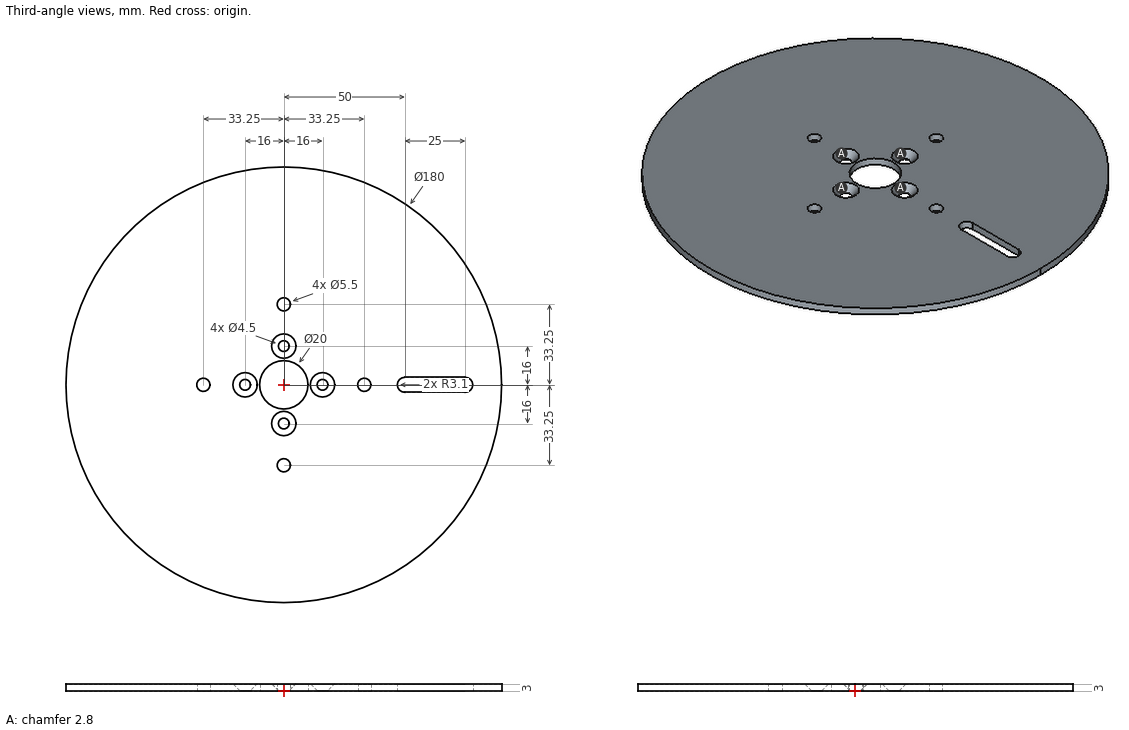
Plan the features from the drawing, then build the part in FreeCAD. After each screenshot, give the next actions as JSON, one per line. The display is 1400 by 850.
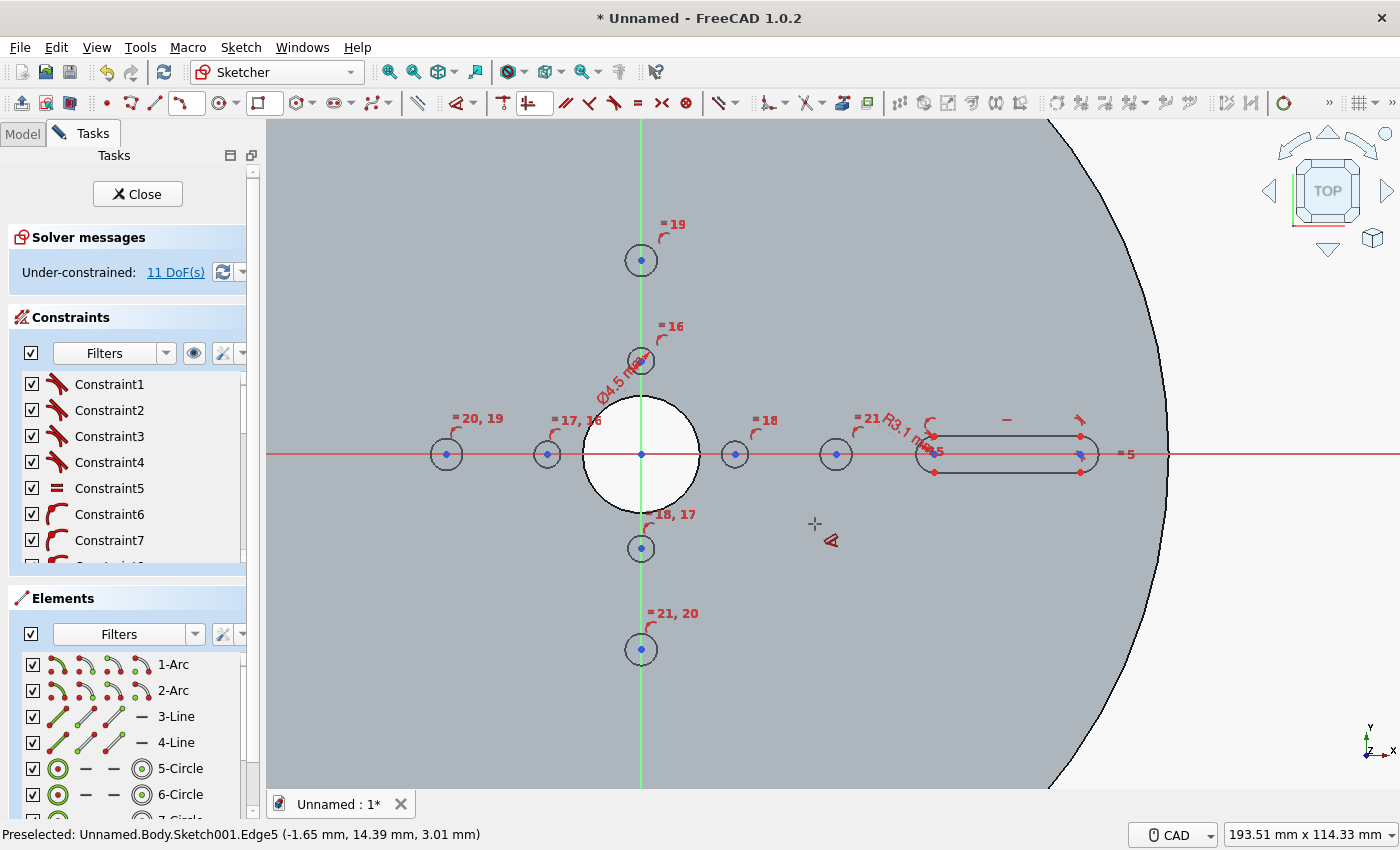
{"action": "scroll", "coordinate": [652, 249], "scroll_direction": "up", "scroll_amount": 2}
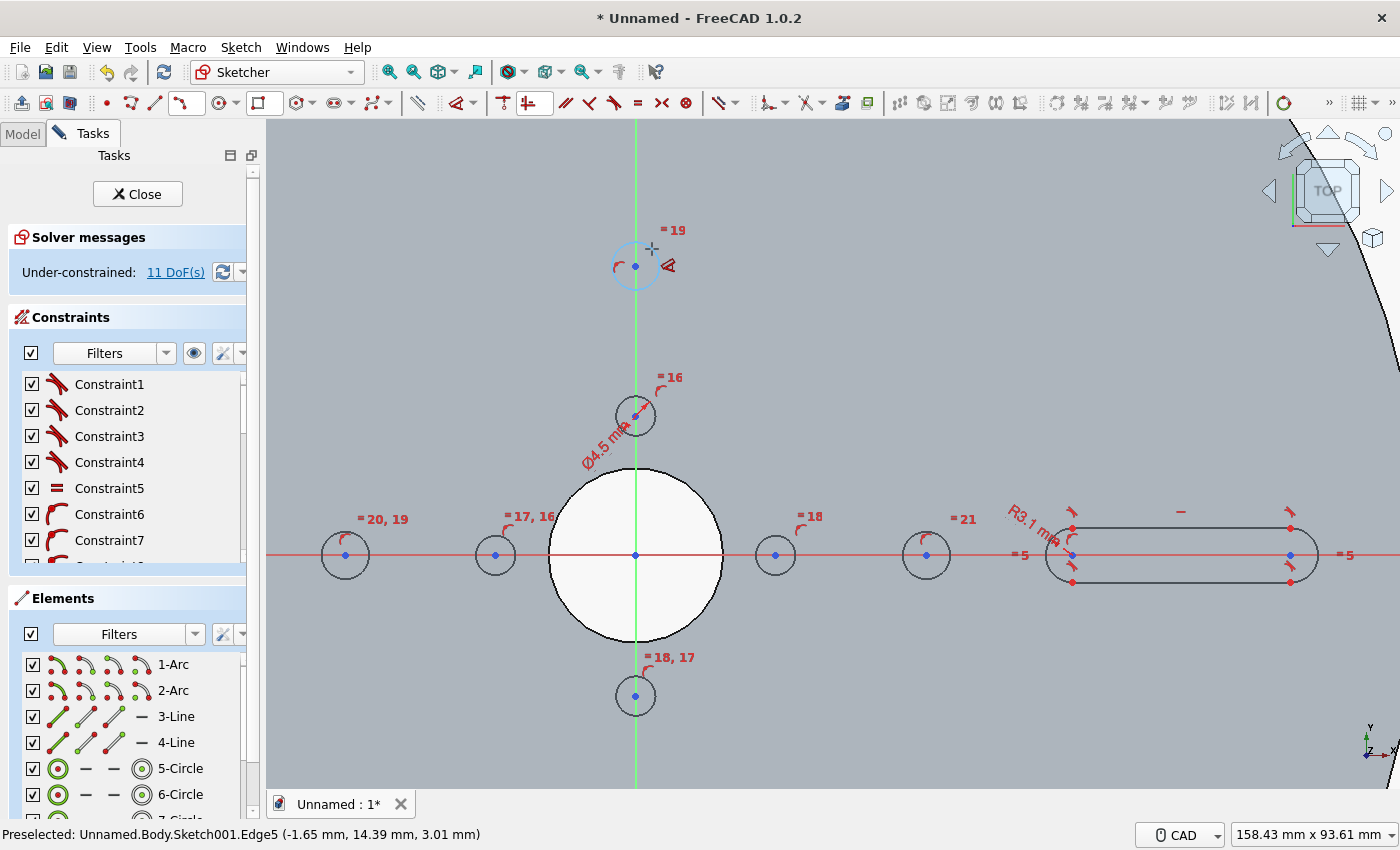
{"action": "left_click", "coordinate": [653, 249]}
{"action": "left_click", "coordinate": [676, 226]}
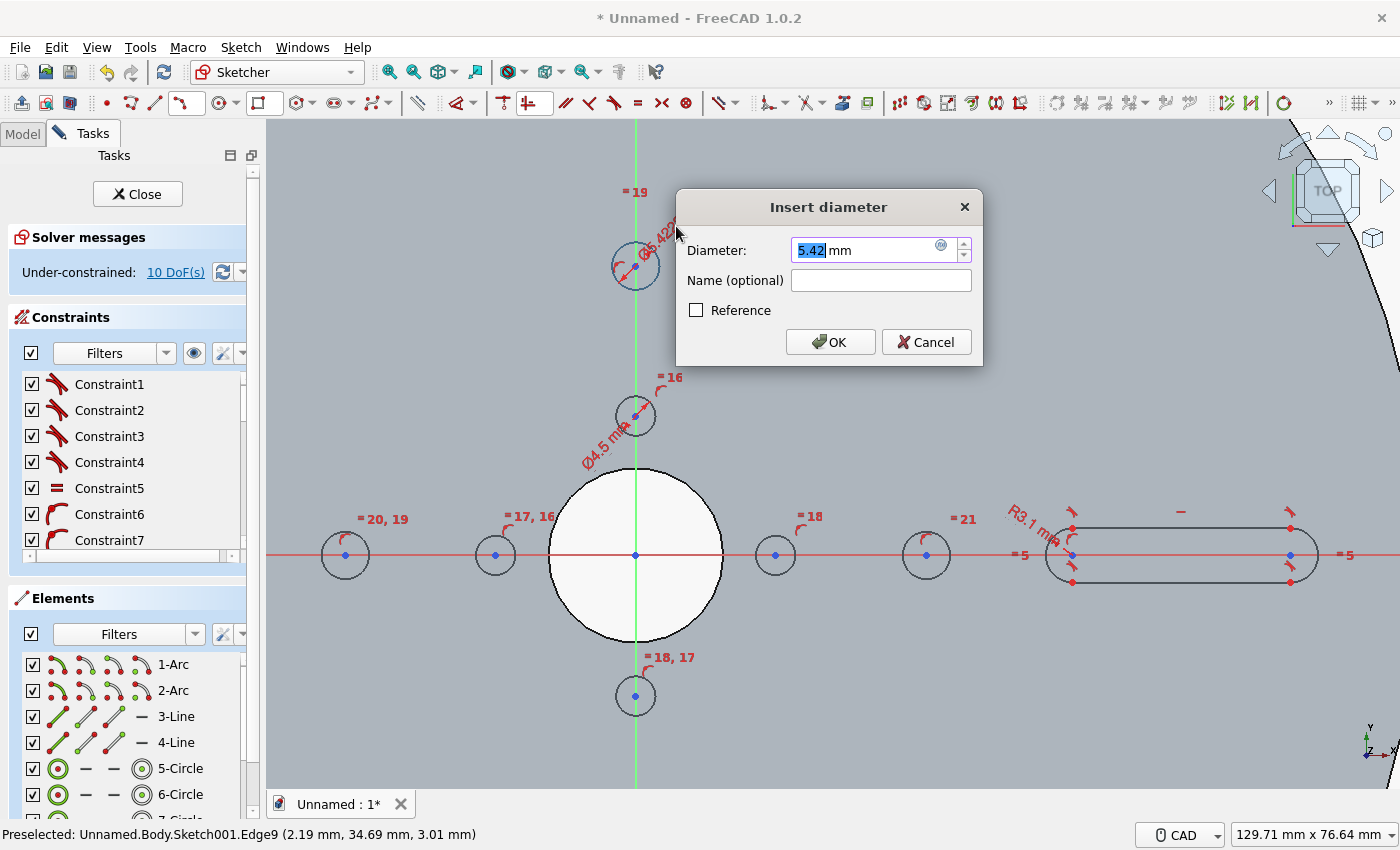
{"action": "type", "text": "5.5"}
{"action": "key", "text": "Return"}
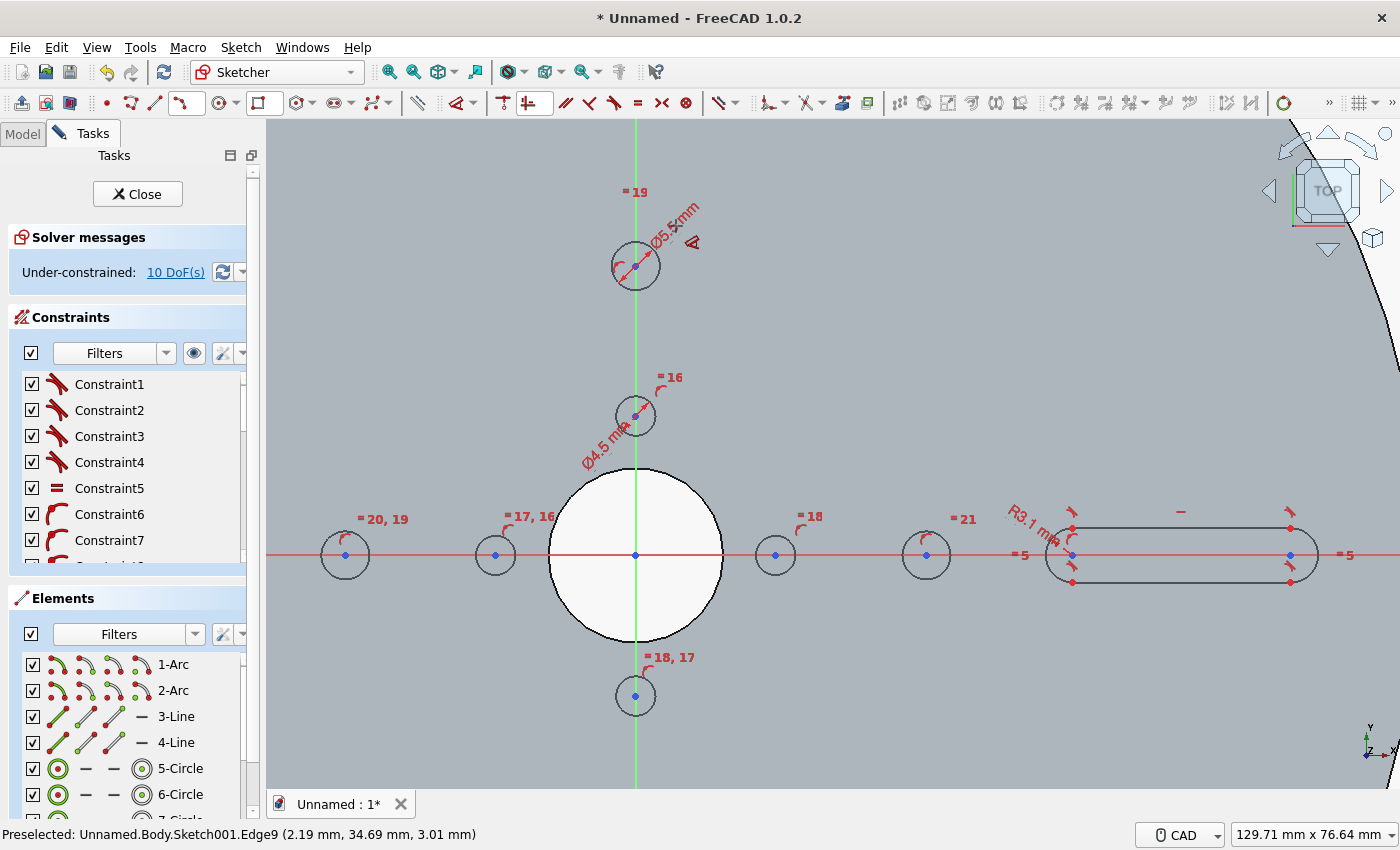
{"action": "left_click", "coordinate": [1138, 528]}
{"action": "left_click", "coordinate": [1154, 494]}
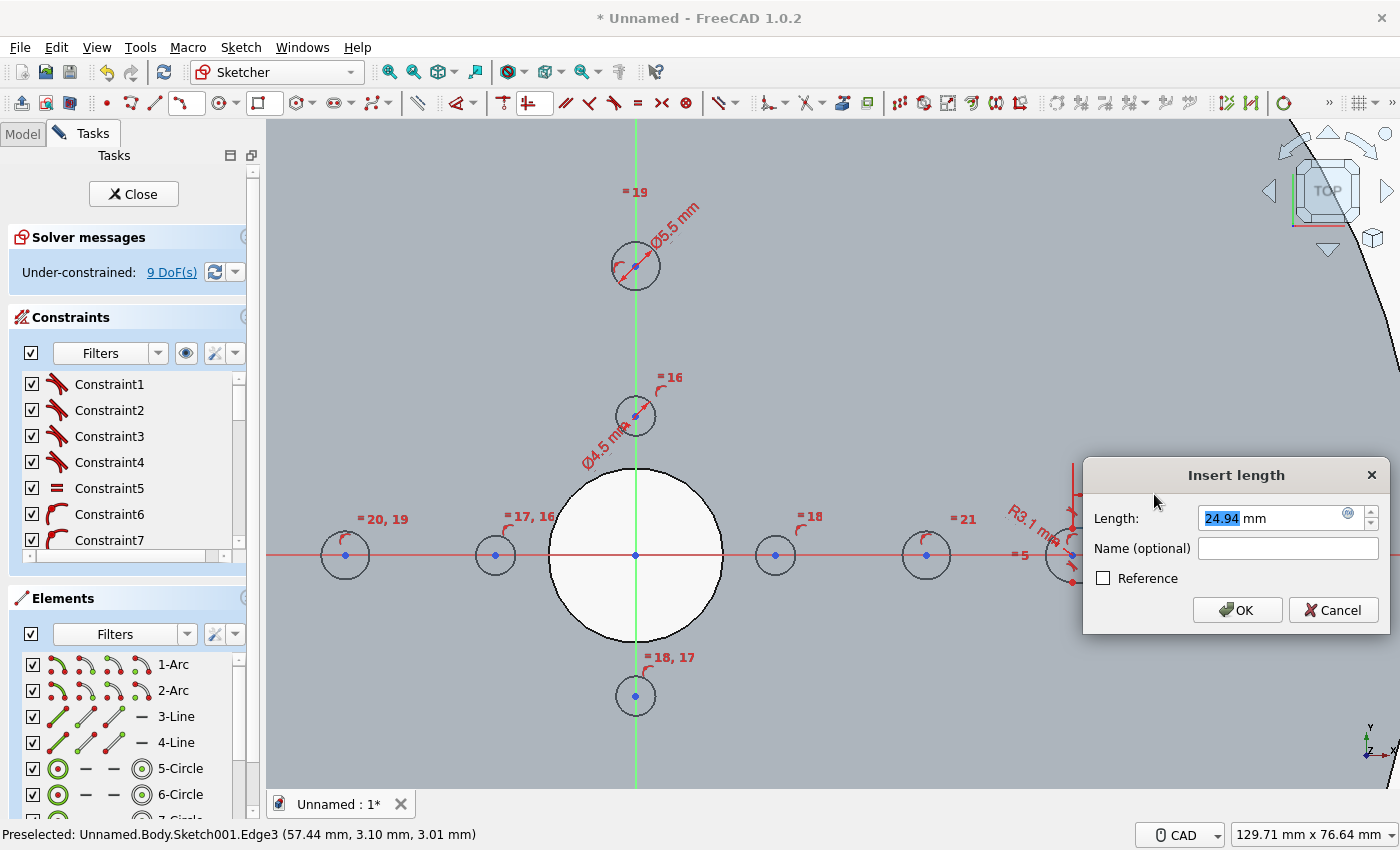
{"action": "type", "text": "25"}
{"action": "key", "text": "Return"}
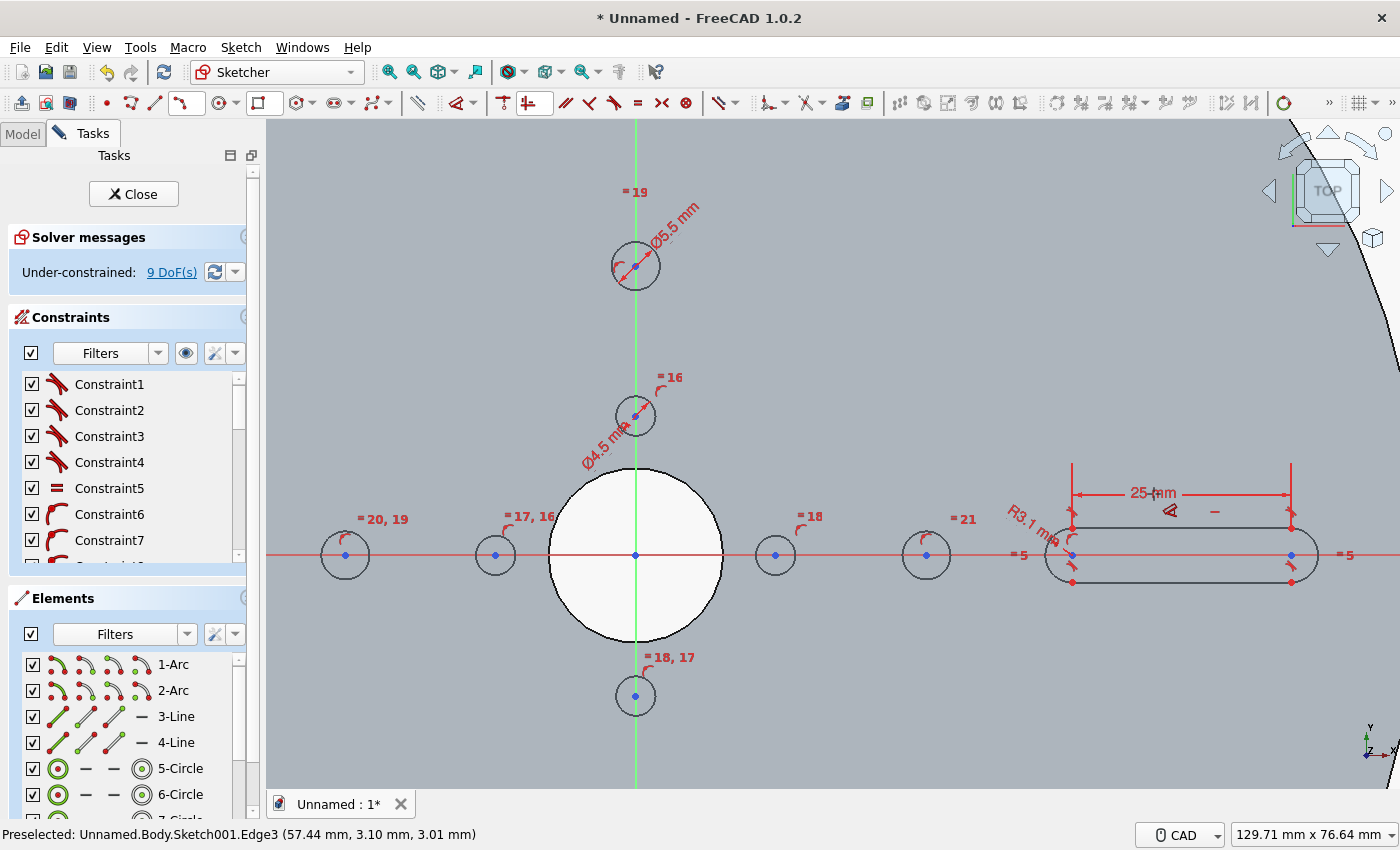
{"action": "left_click", "coordinate": [636, 416]}
{"action": "left_click", "coordinate": [602, 486]}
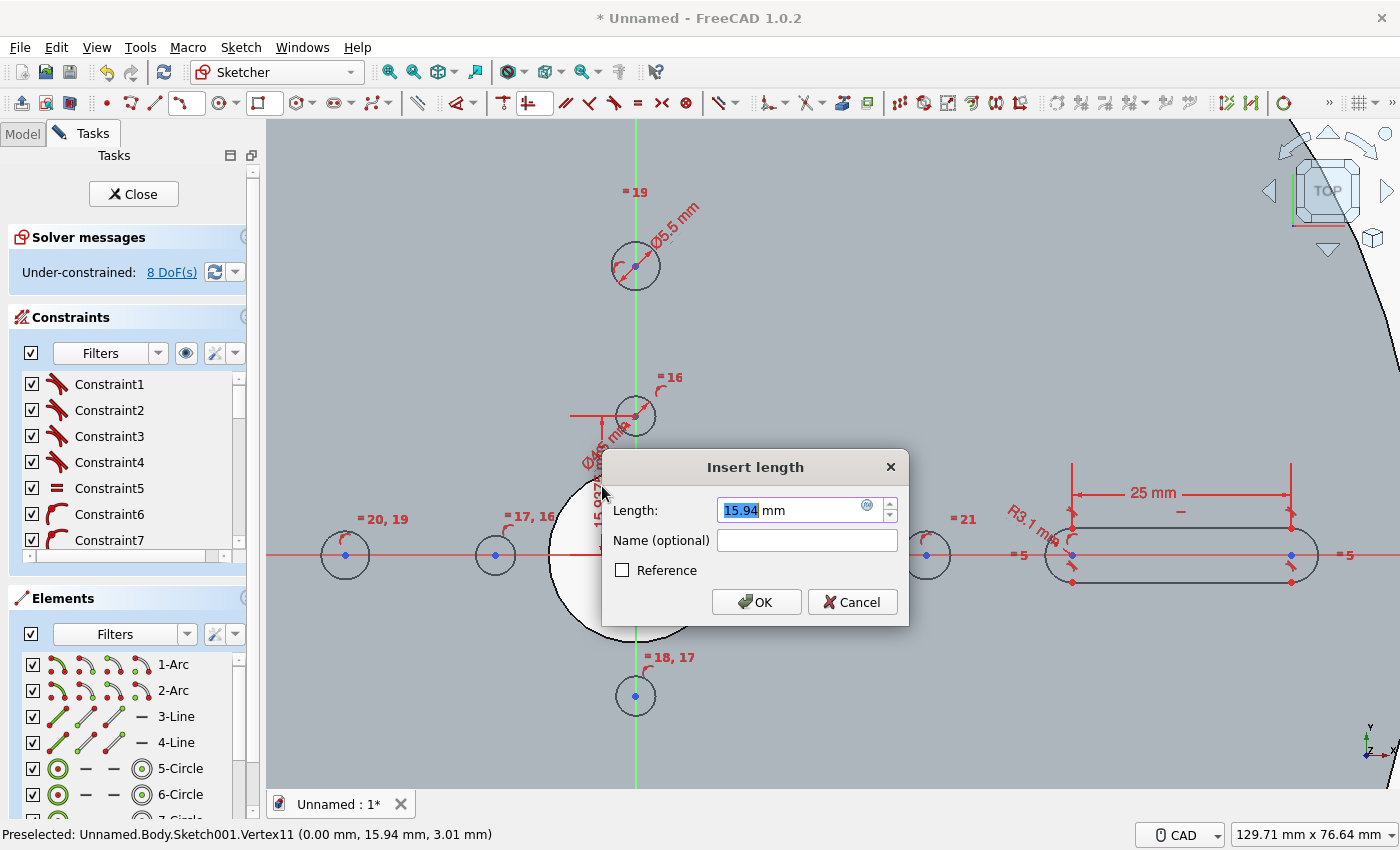
{"action": "type", "text": "16"}
{"action": "key", "text": "Return"}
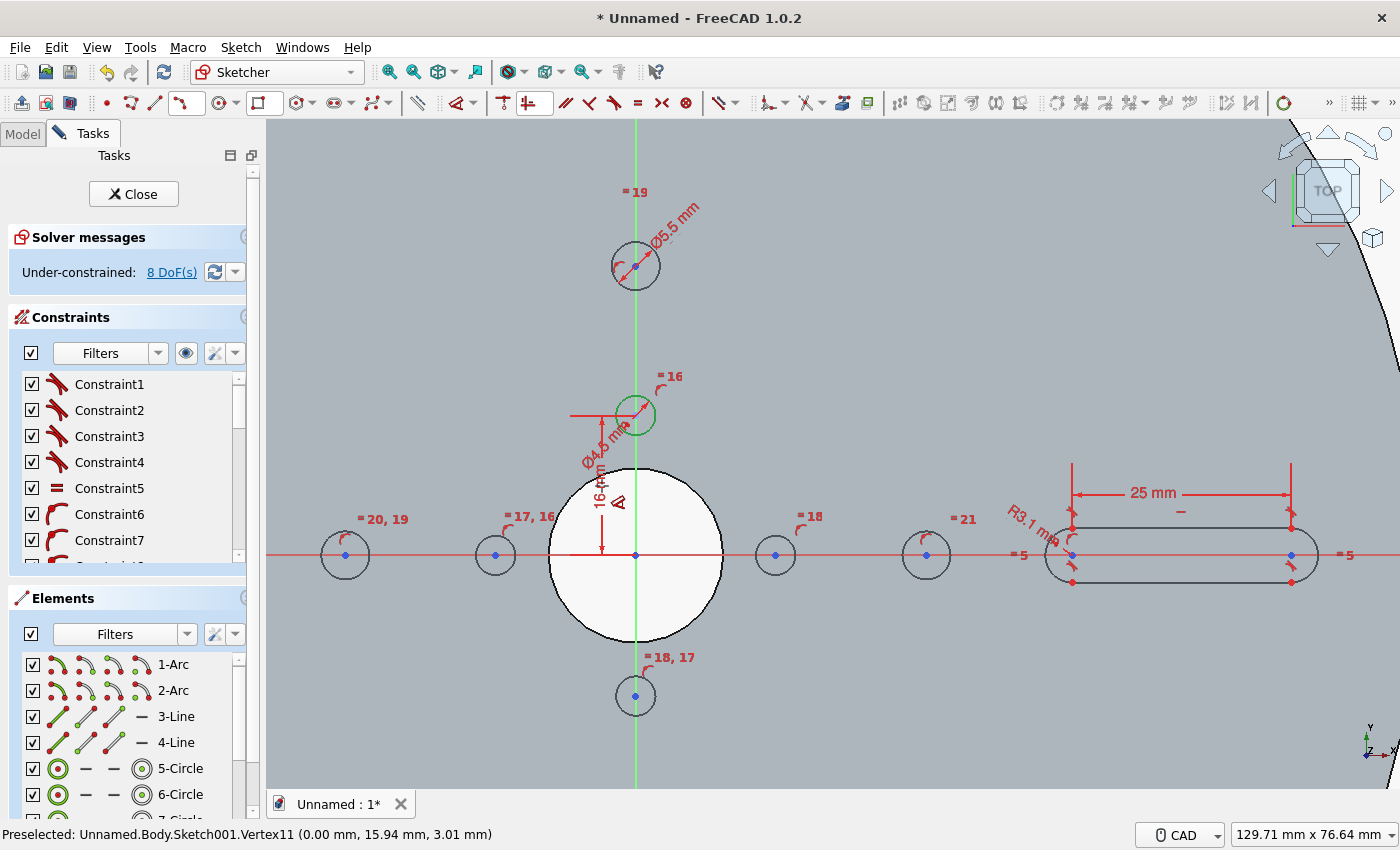
{"action": "left_click", "coordinate": [496, 555]}
{"action": "left_click", "coordinate": [566, 589]}